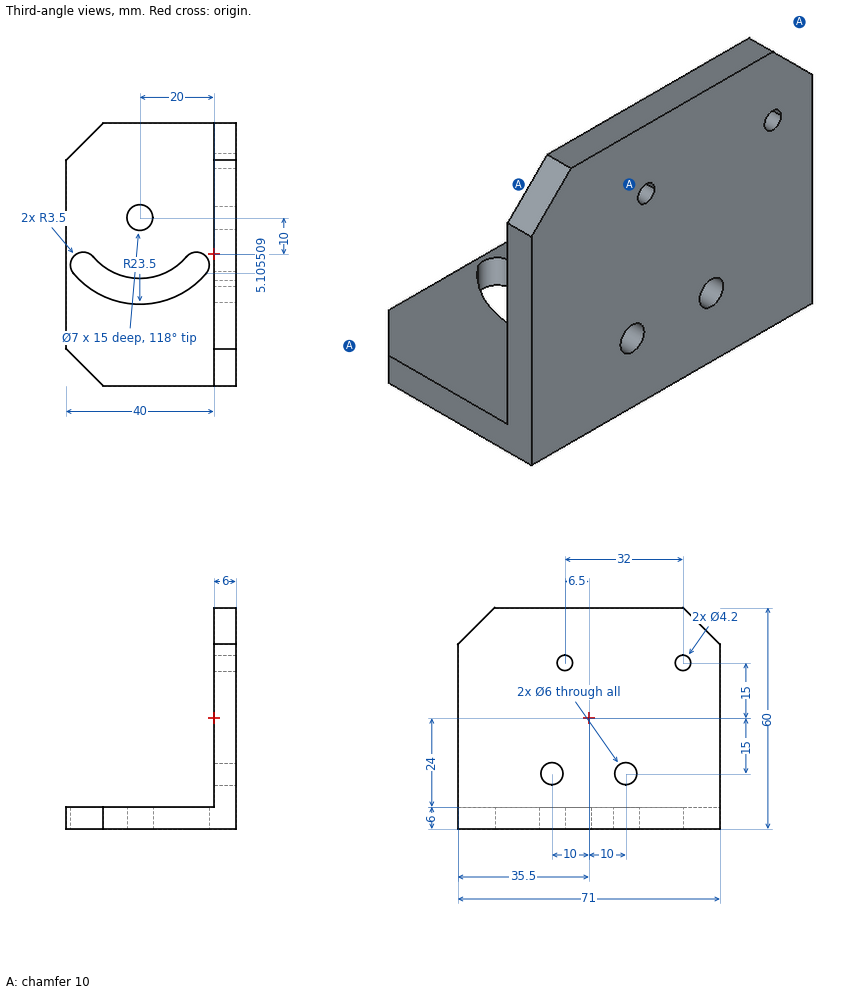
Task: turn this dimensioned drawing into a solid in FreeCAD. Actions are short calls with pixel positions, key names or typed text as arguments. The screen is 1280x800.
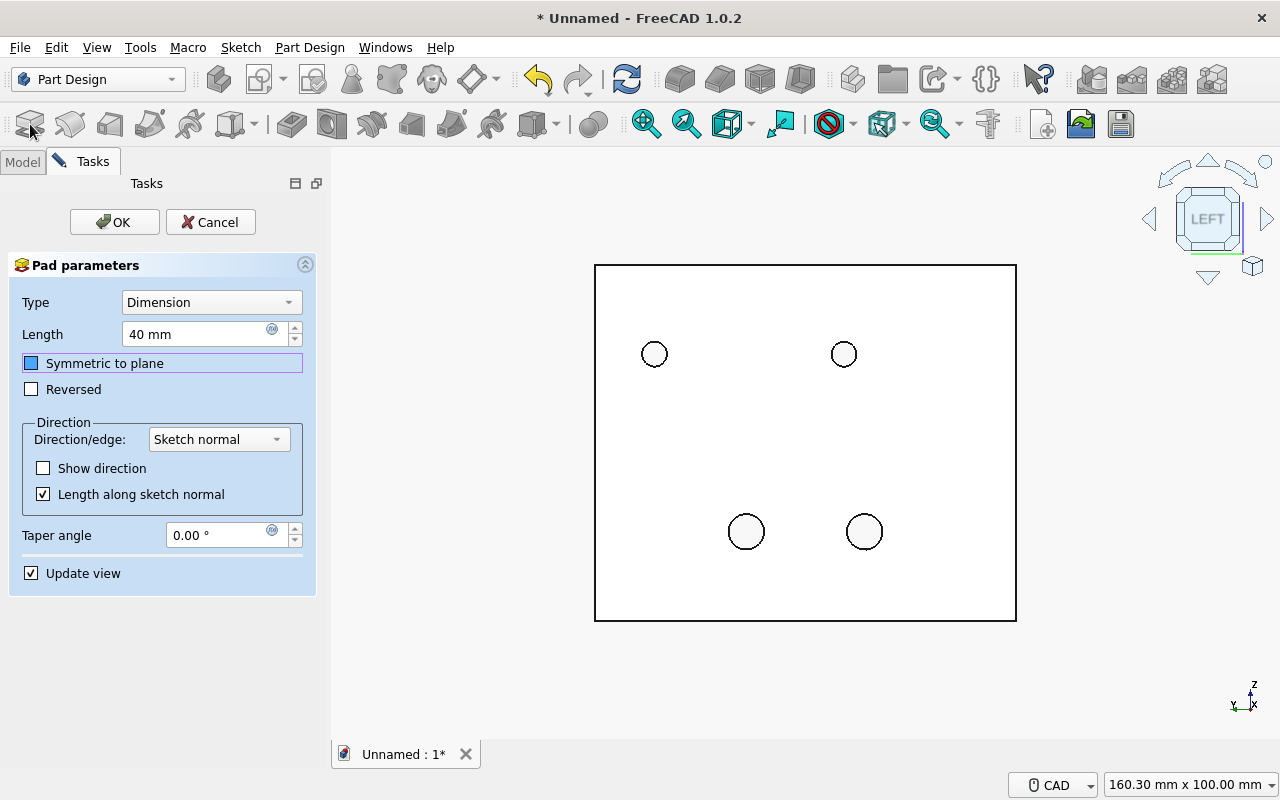
click(30, 389)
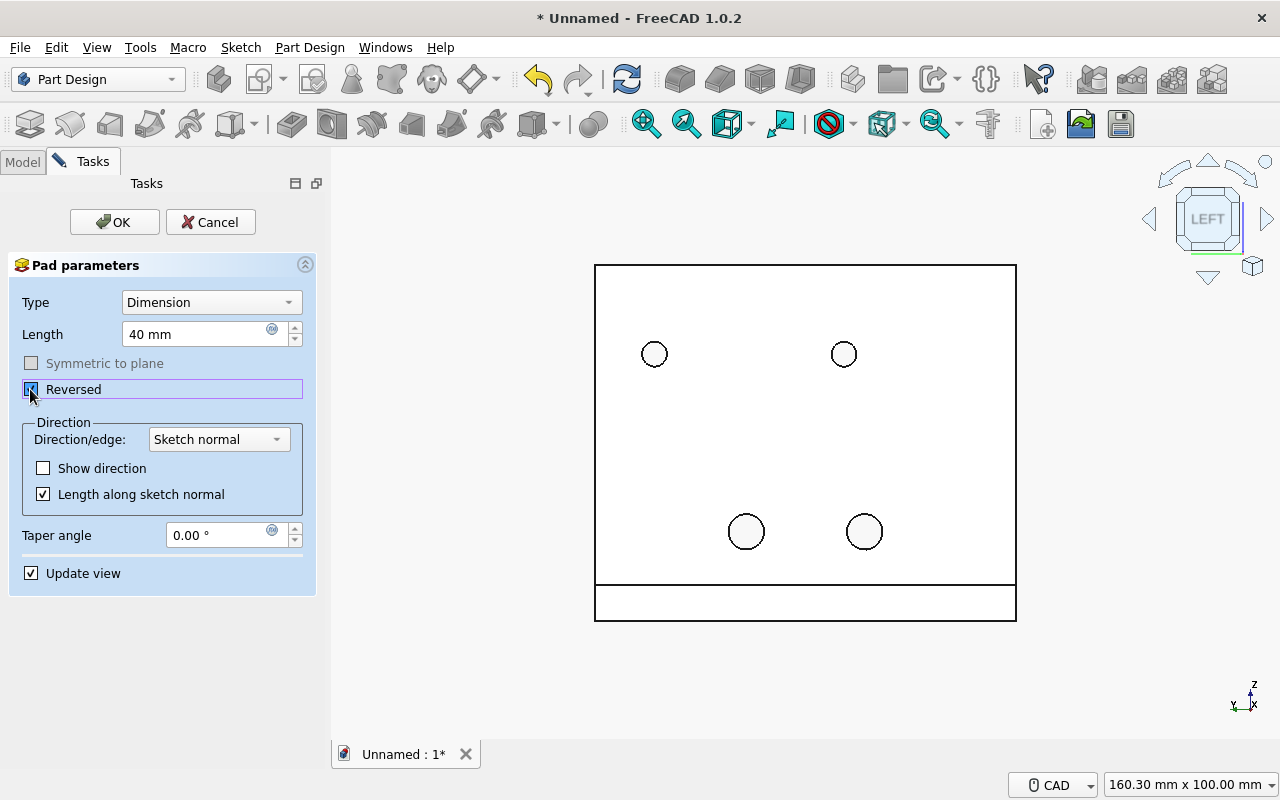
click(115, 222)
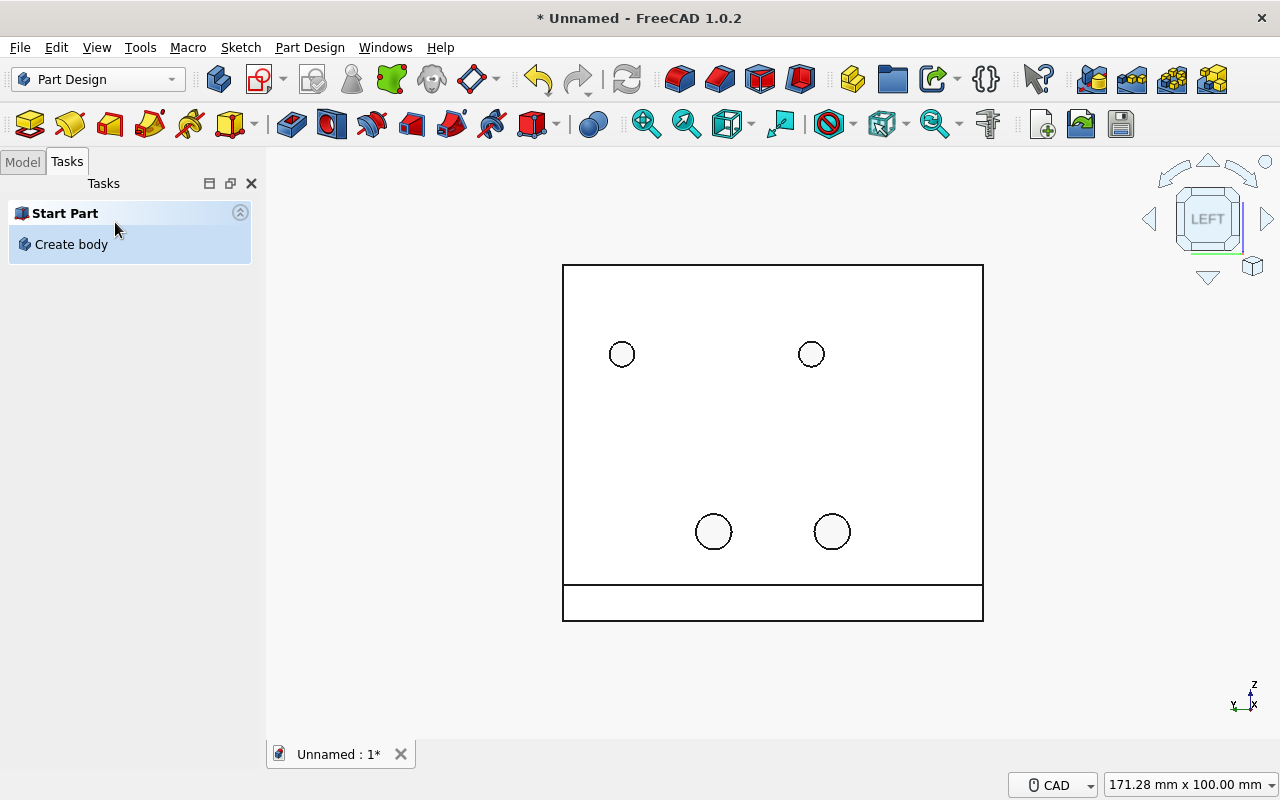
key(5)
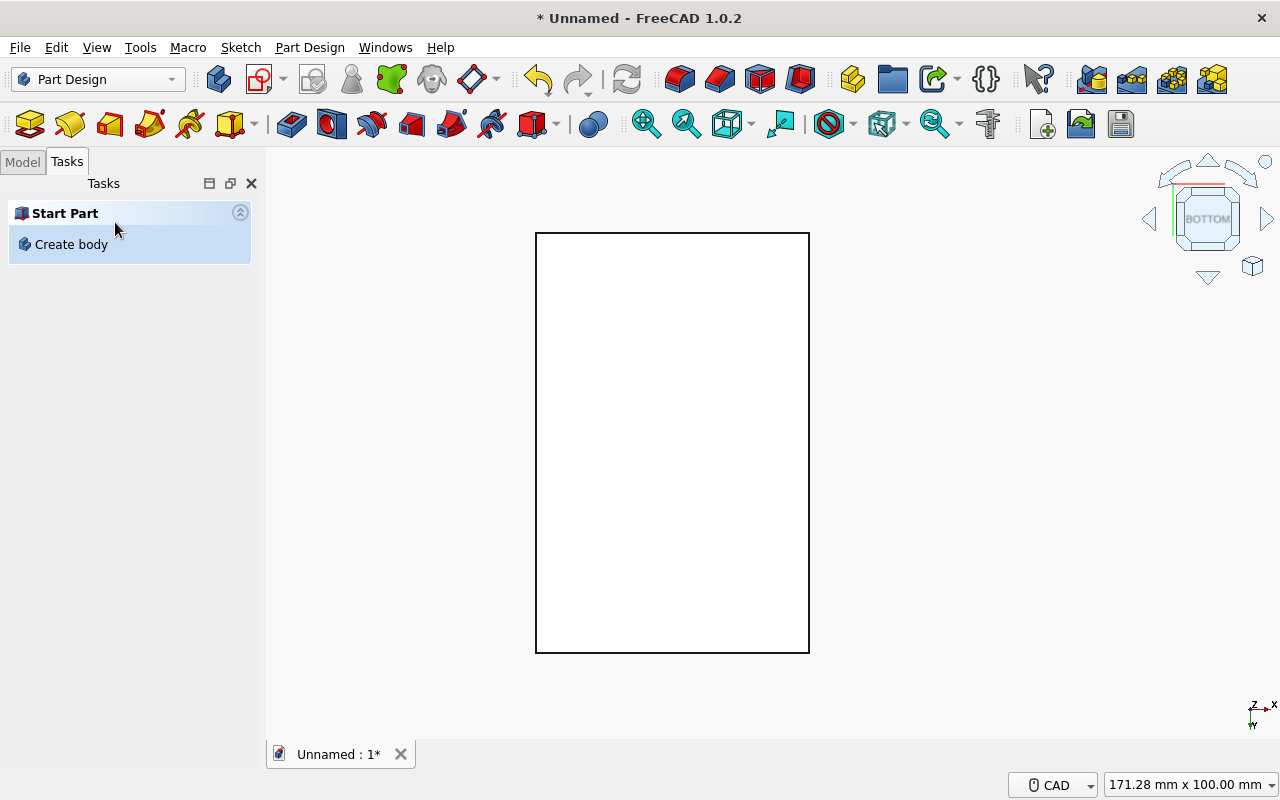
click(672, 502)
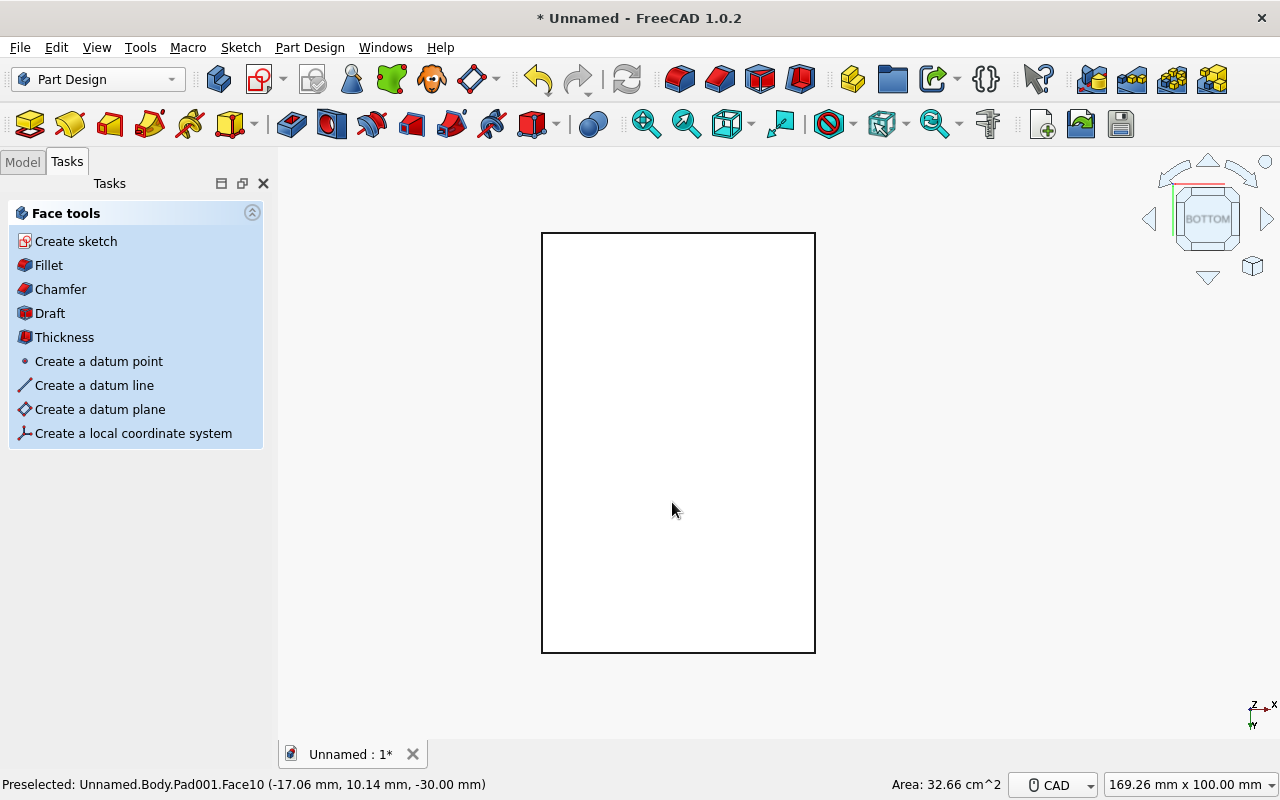
click(260, 80)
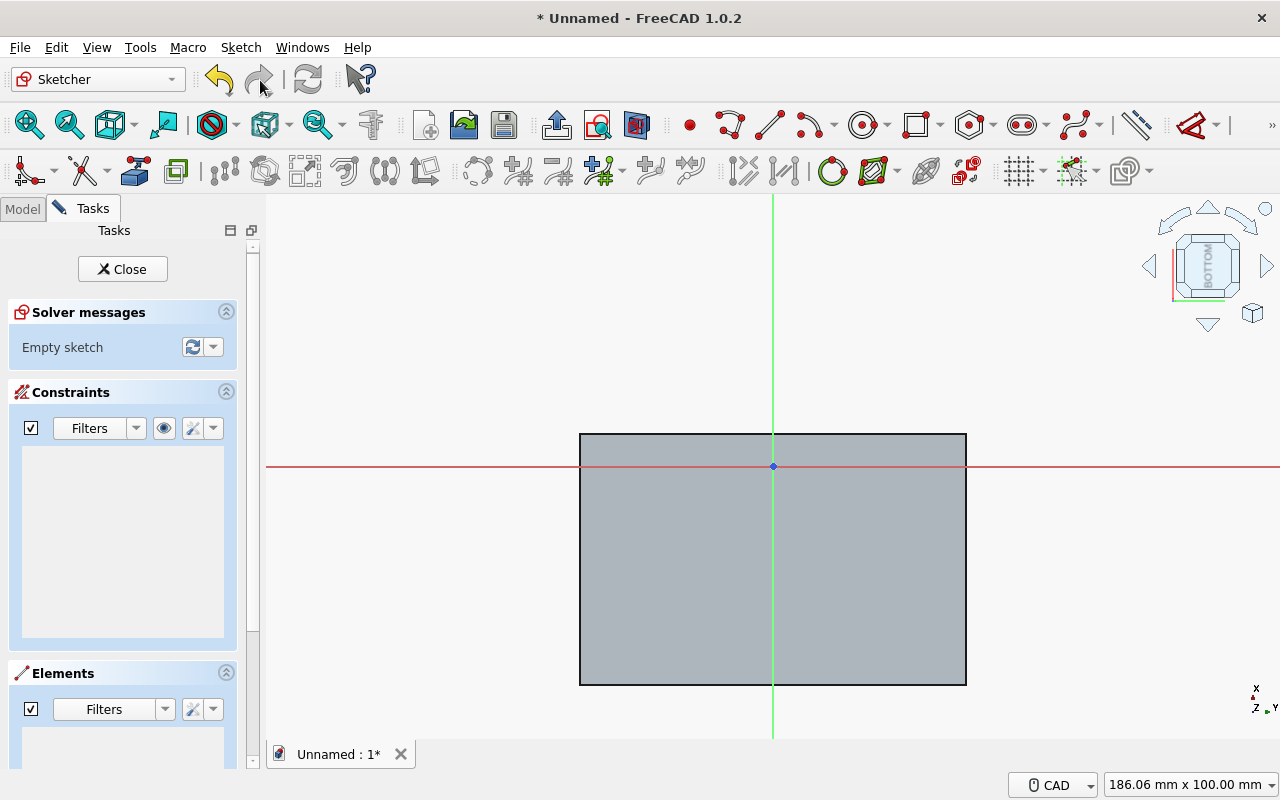
scroll(843, 589, up, 11)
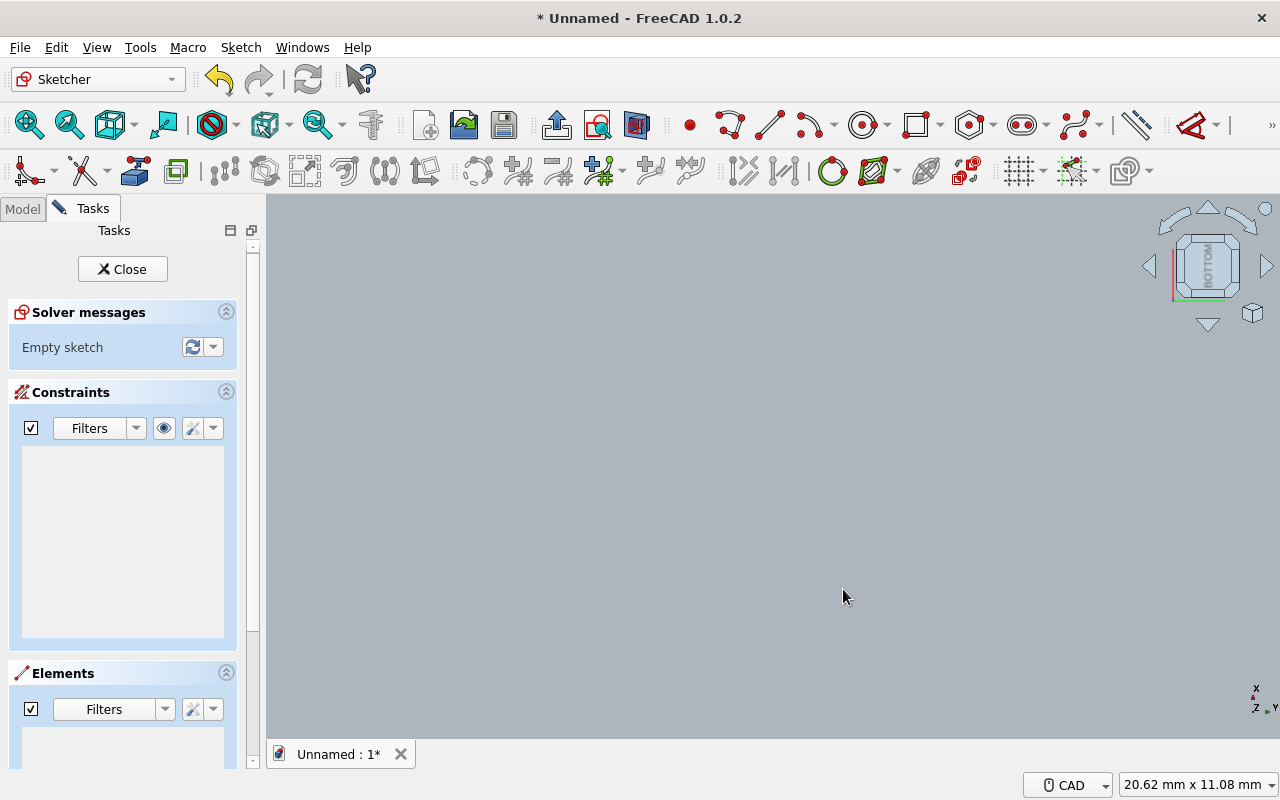
click(864, 126)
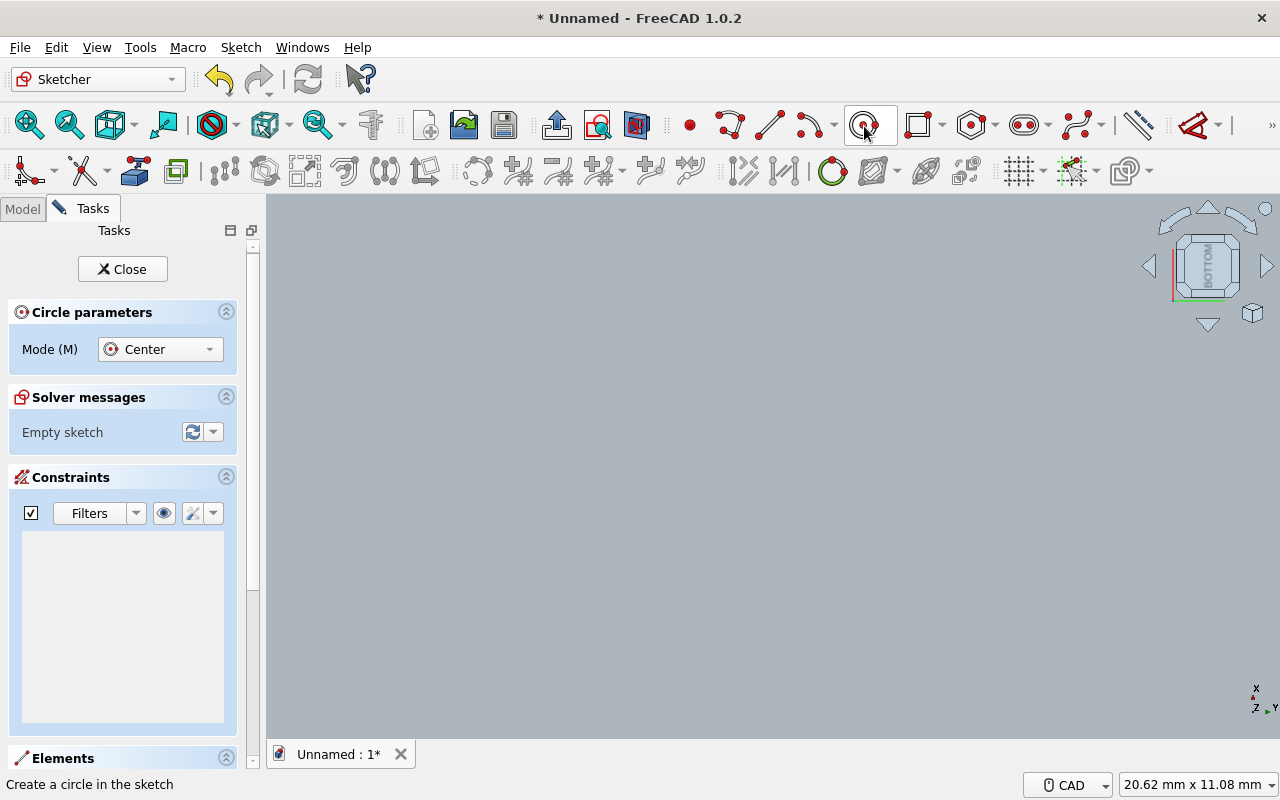
click(699, 461)
click(820, 340)
key(Escape)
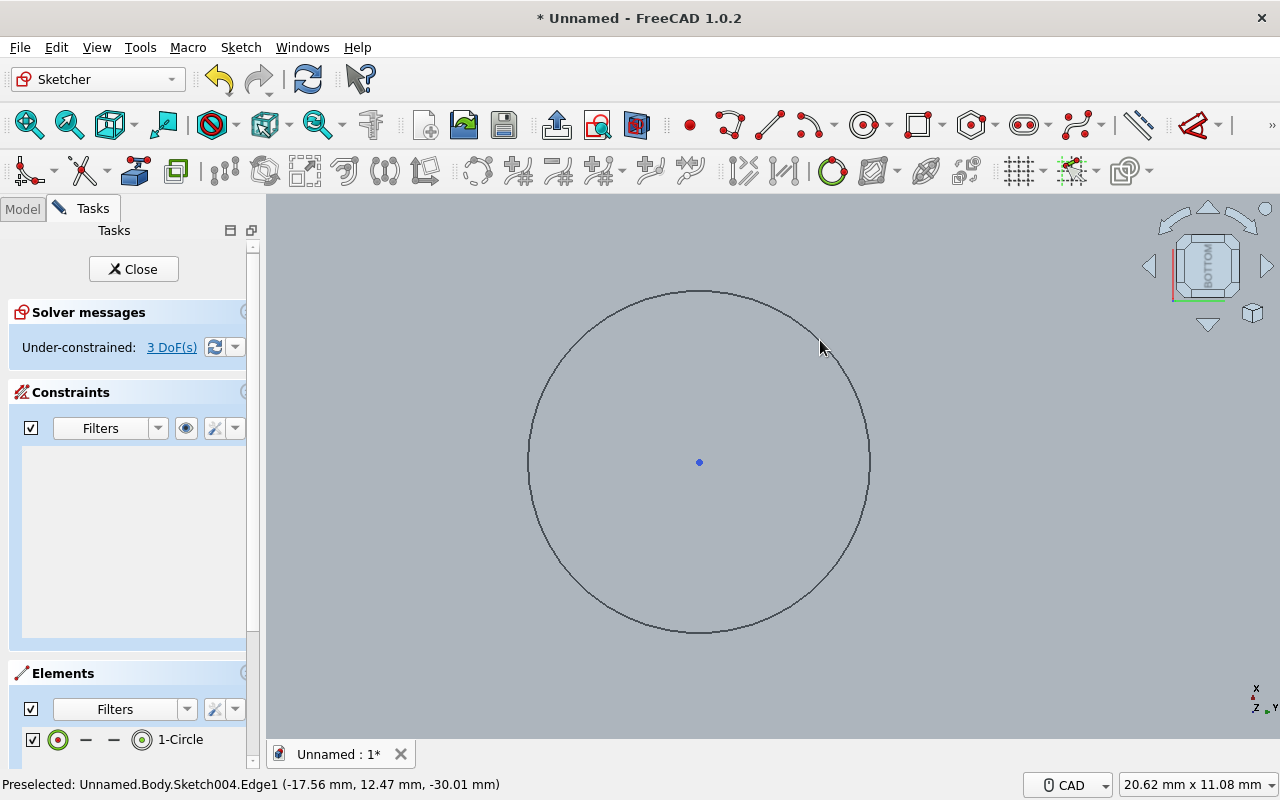
click(1194, 126)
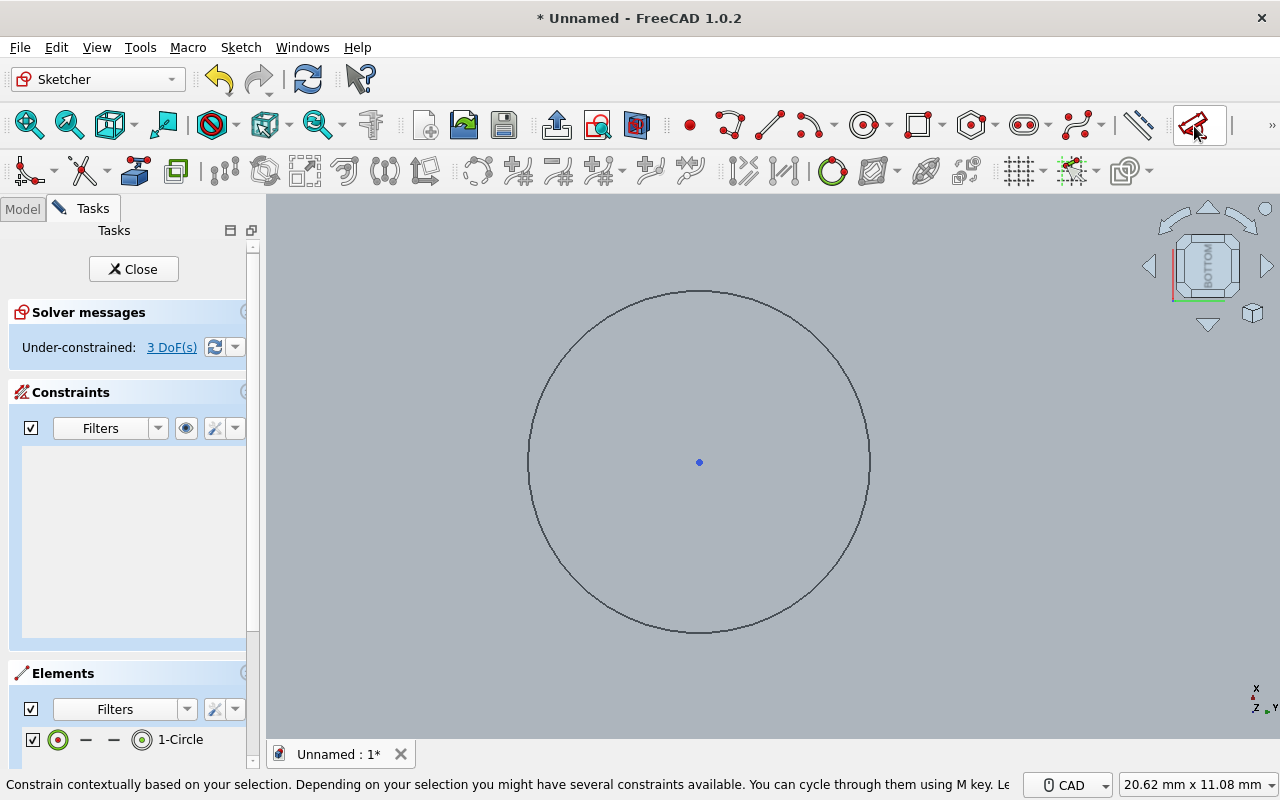
click(820, 341)
click(843, 318)